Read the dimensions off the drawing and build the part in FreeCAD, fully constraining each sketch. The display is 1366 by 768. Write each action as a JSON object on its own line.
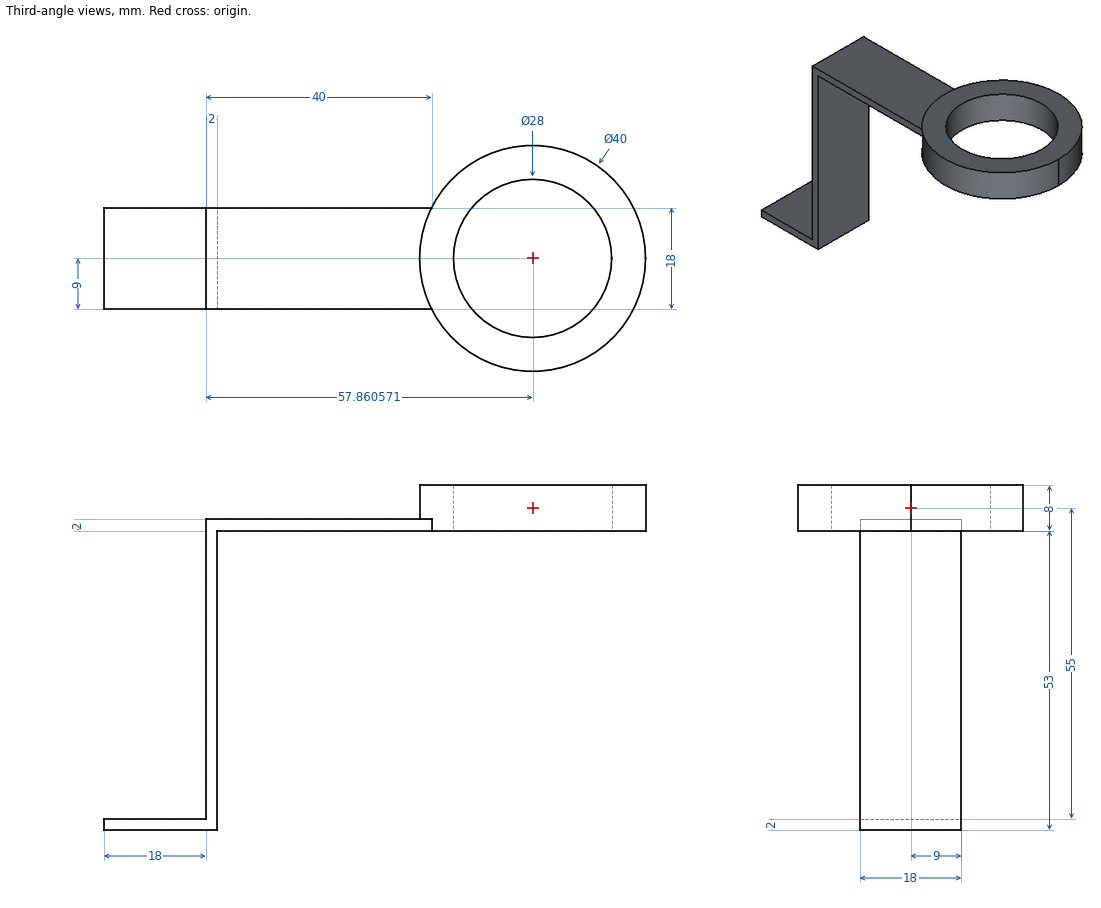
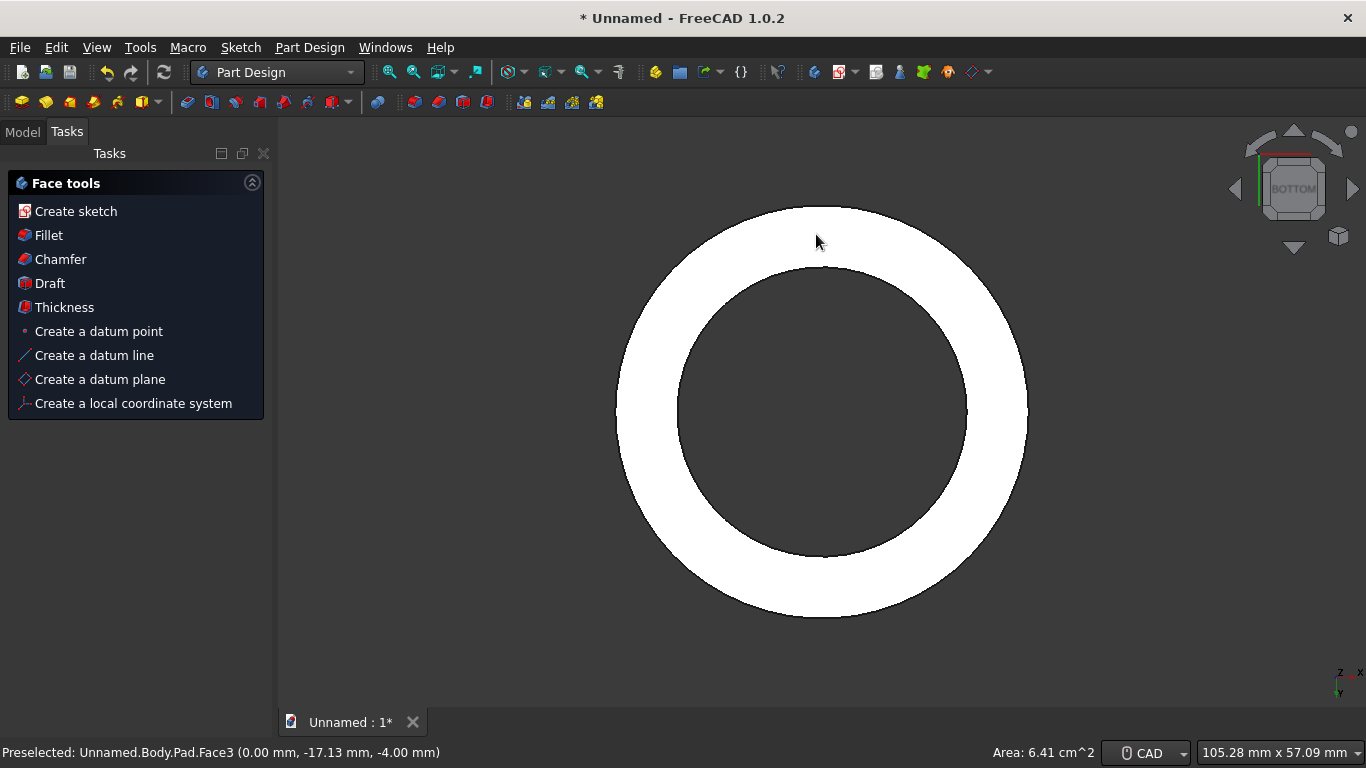
{"action": "left_click", "coordinate": [840, 72]}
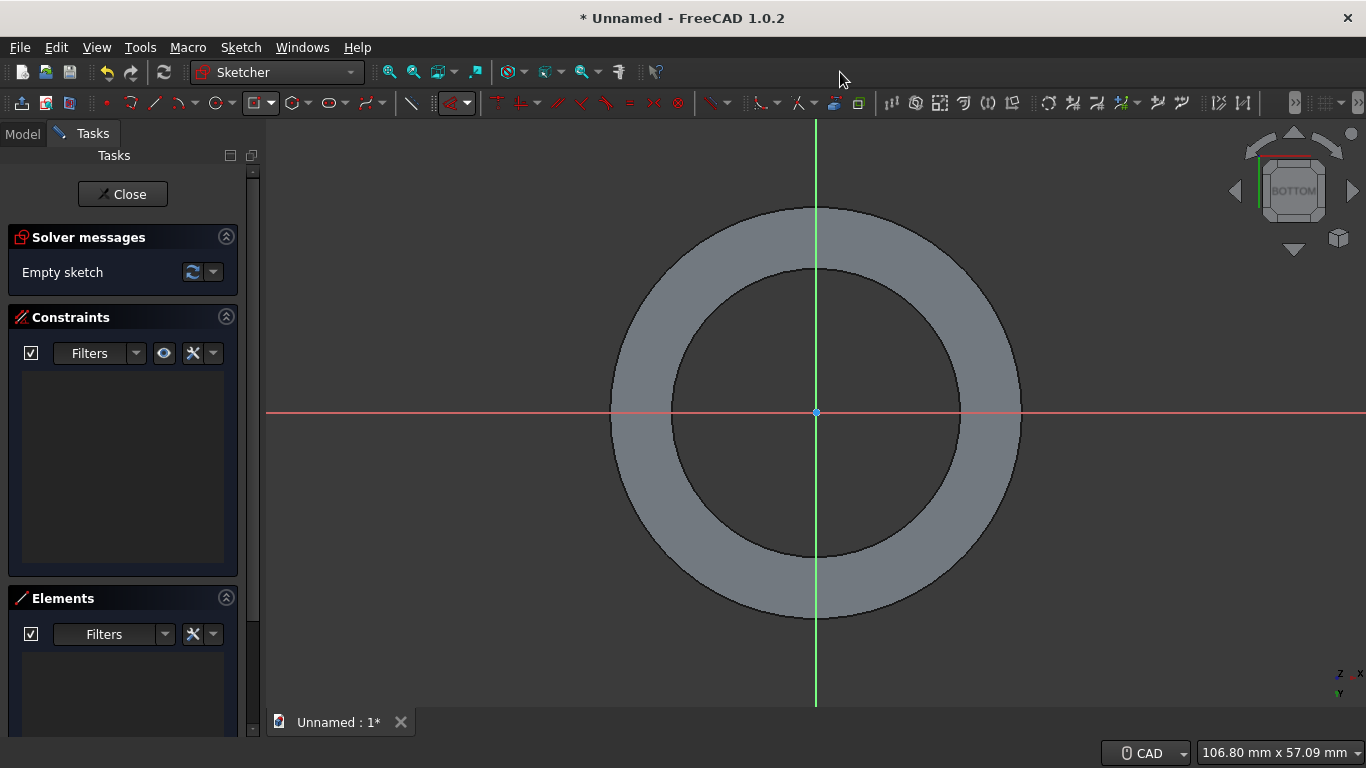
{"action": "scroll", "coordinate": [1201, 413], "scroll_direction": "down", "scroll_amount": 1}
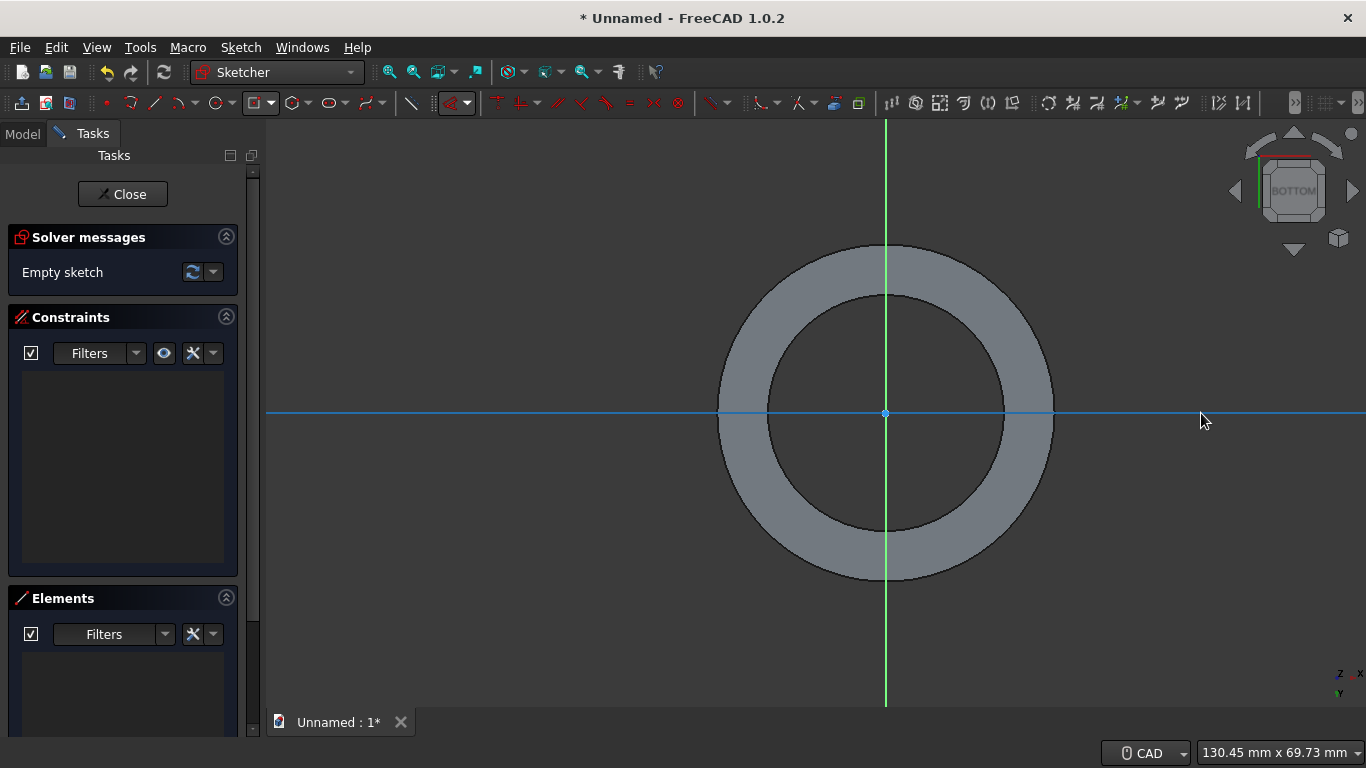
{"action": "key", "text": "g r"}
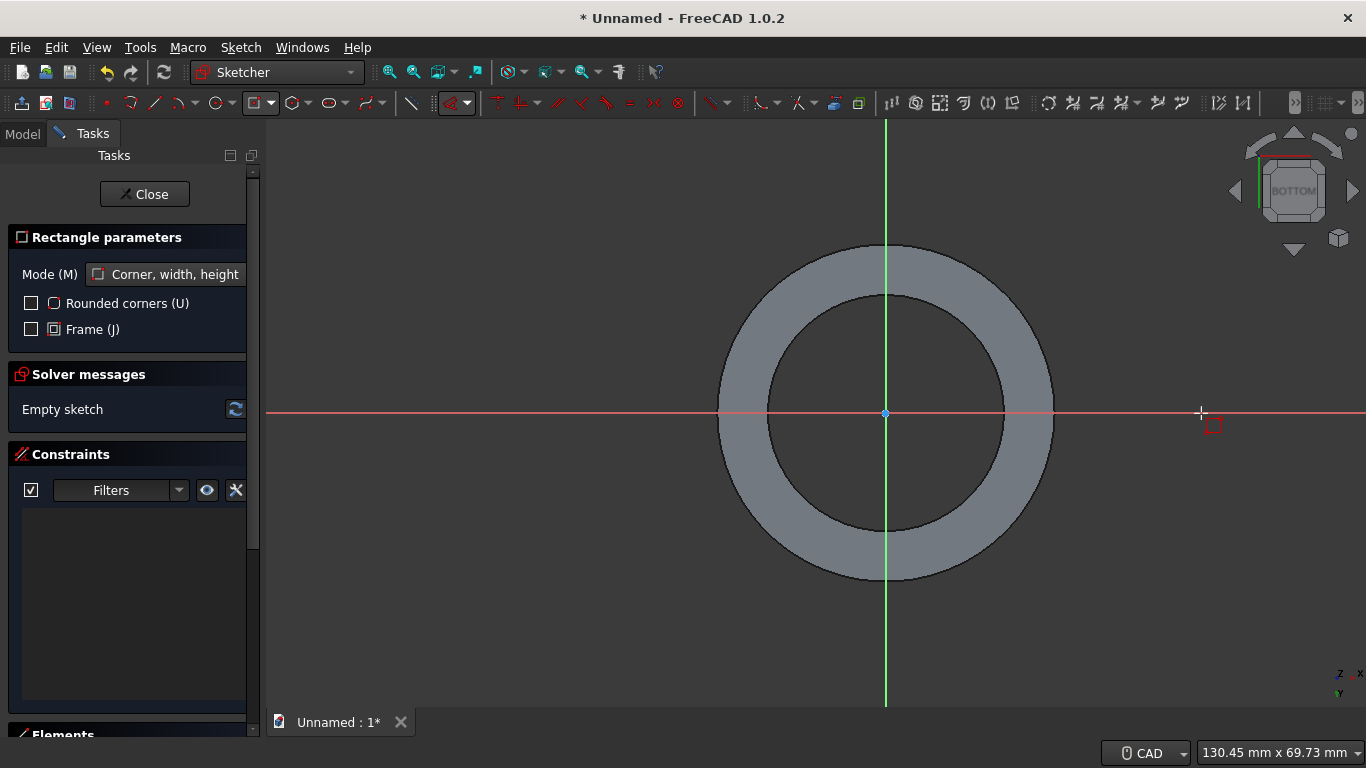
{"action": "left_click", "coordinate": [398, 337]}
{"action": "mouse_move", "coordinate": [735, 489]}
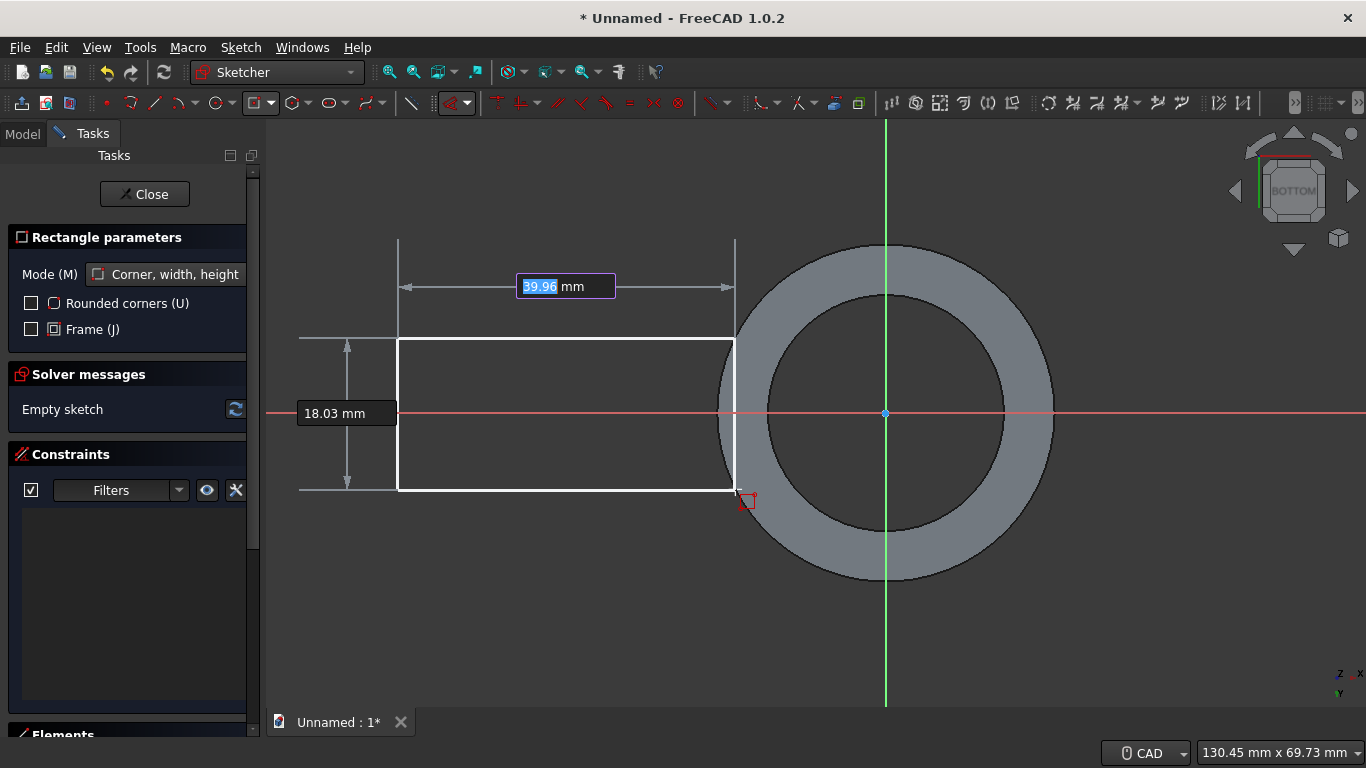
{"action": "type", "text": "40"}
{"action": "key", "text": "Tab"}
{"action": "type", "text": "18"}
{"action": "key", "text": "Return"}
{"action": "key", "text": "Escape"}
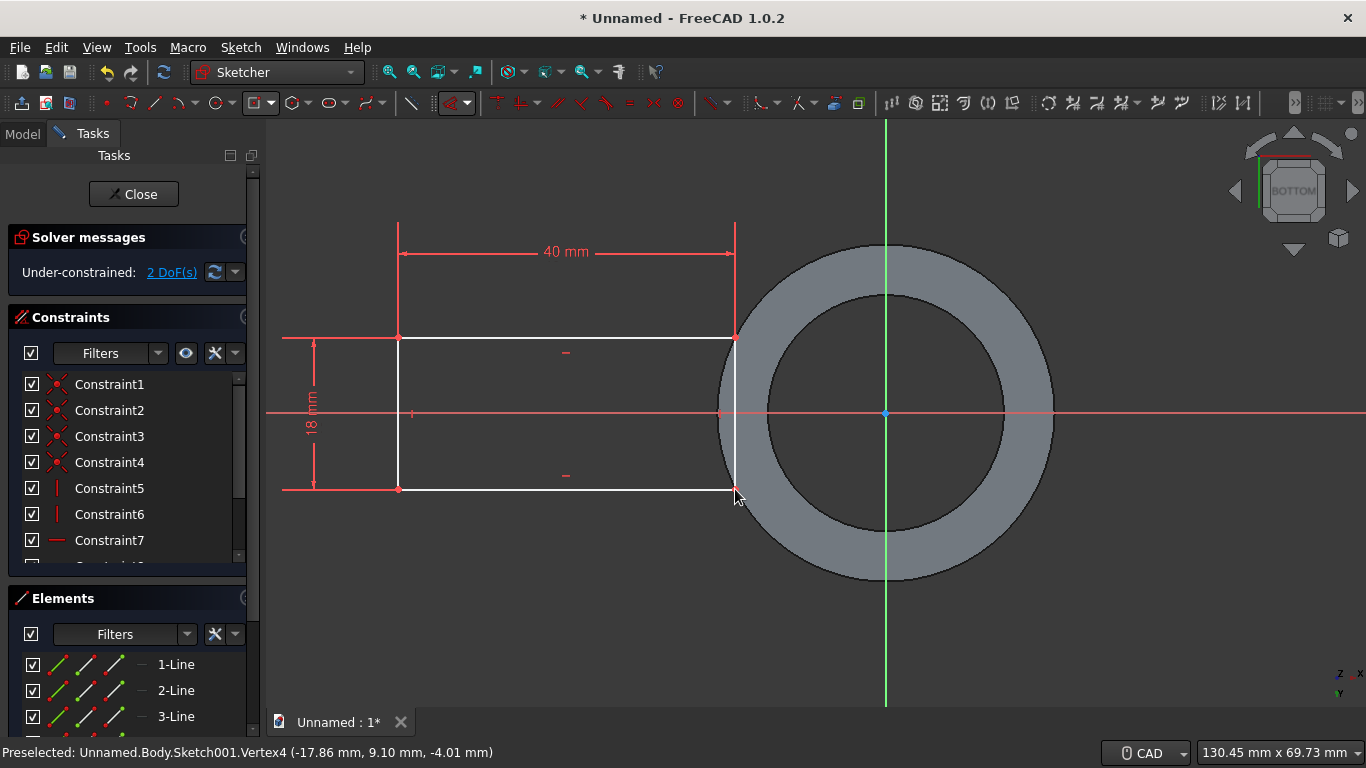
{"action": "left_click", "coordinate": [450, 104]}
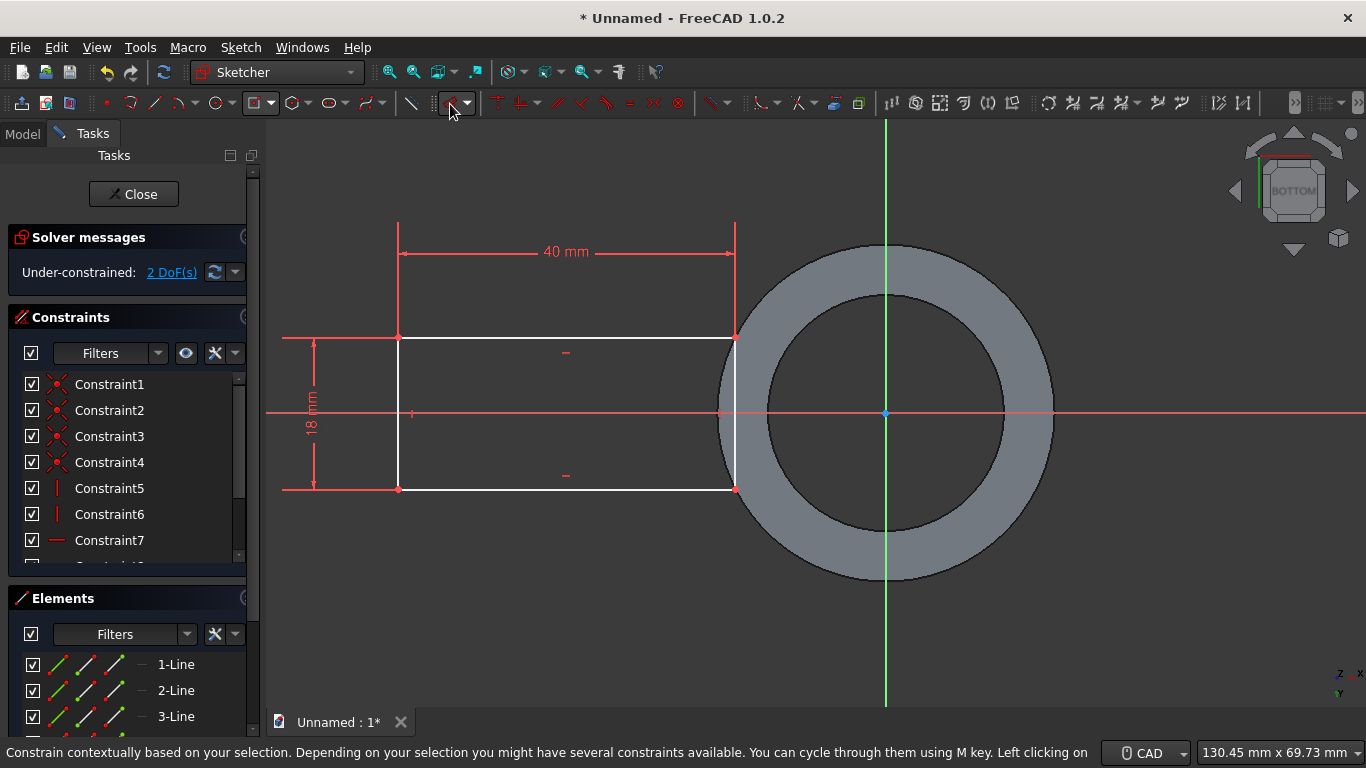
{"action": "left_click", "coordinate": [398, 338]}
{"action": "left_click", "coordinate": [364, 376]}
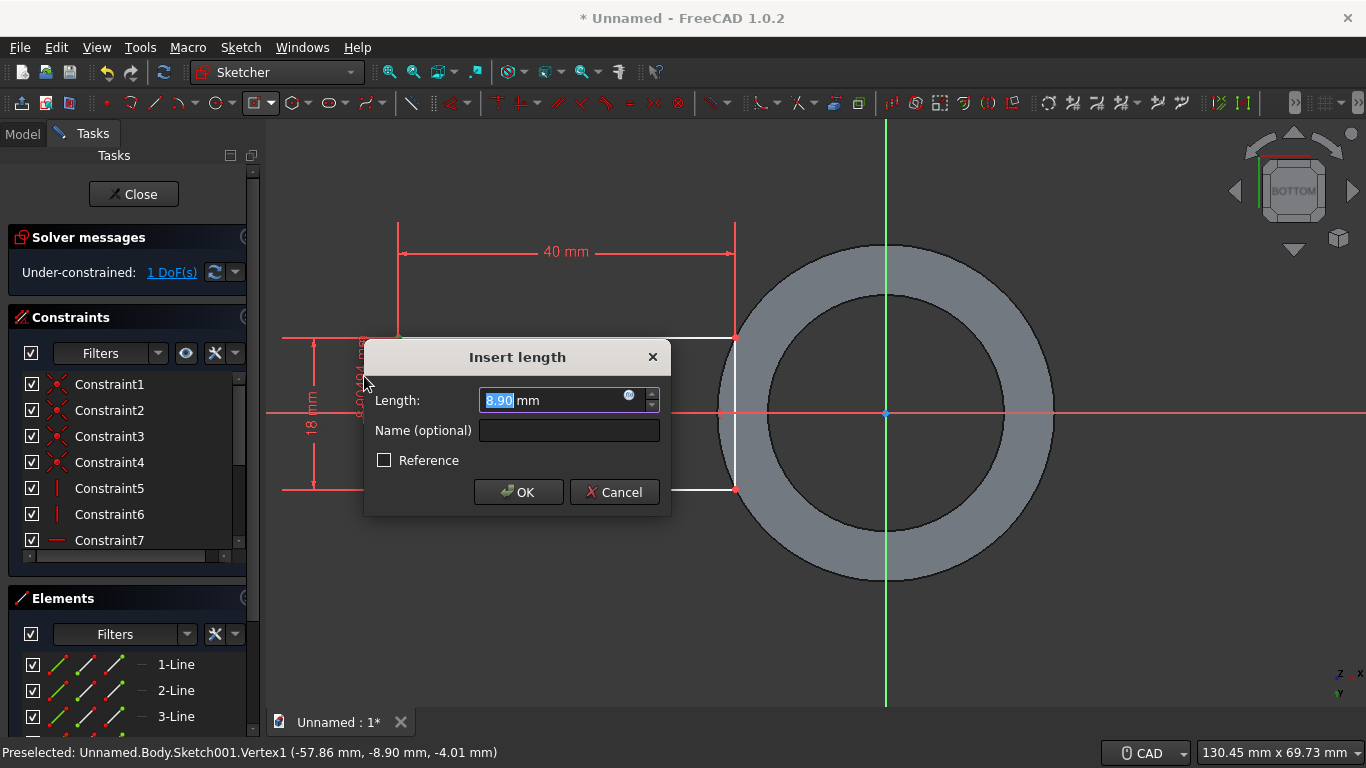
{"action": "type", "text": "9"}
{"action": "key", "text": "Return"}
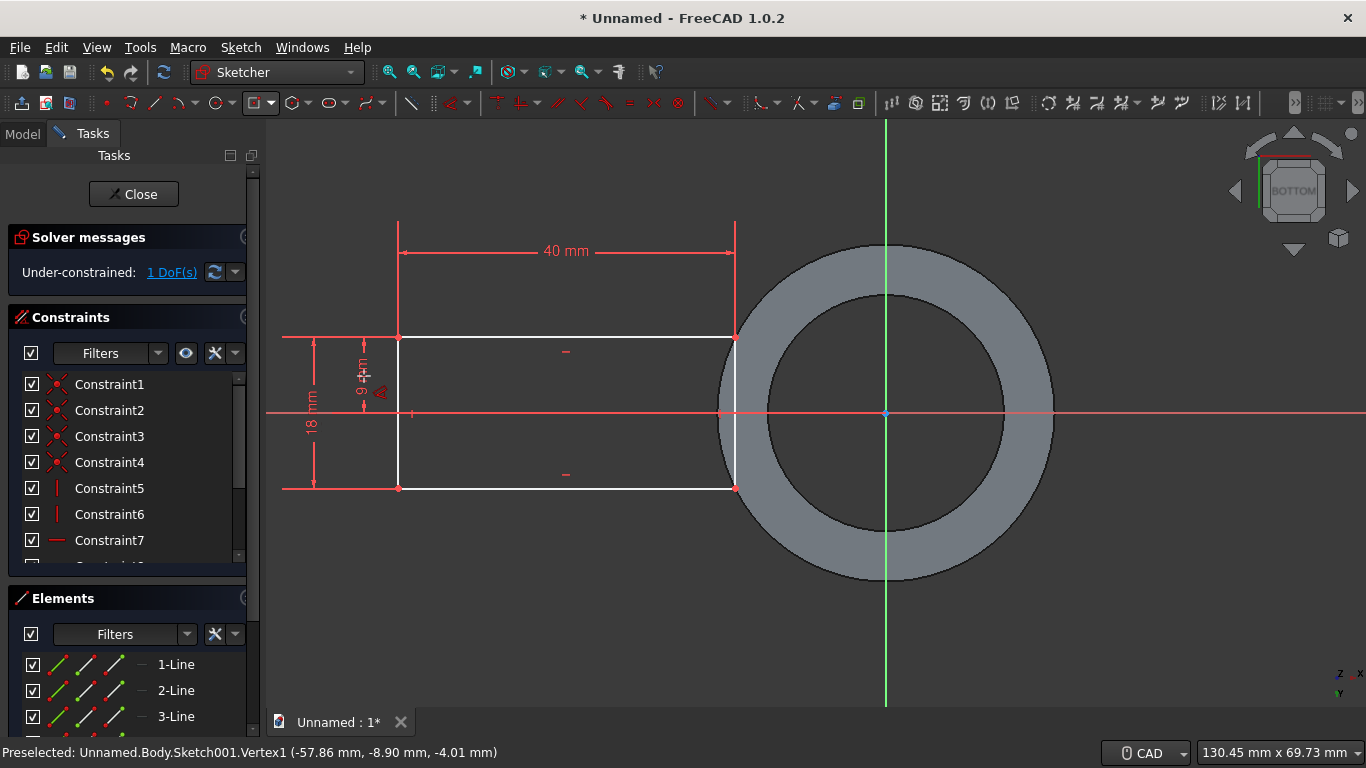
{"action": "left_click", "coordinate": [398, 337]}
{"action": "left_click", "coordinate": [642, 303]}